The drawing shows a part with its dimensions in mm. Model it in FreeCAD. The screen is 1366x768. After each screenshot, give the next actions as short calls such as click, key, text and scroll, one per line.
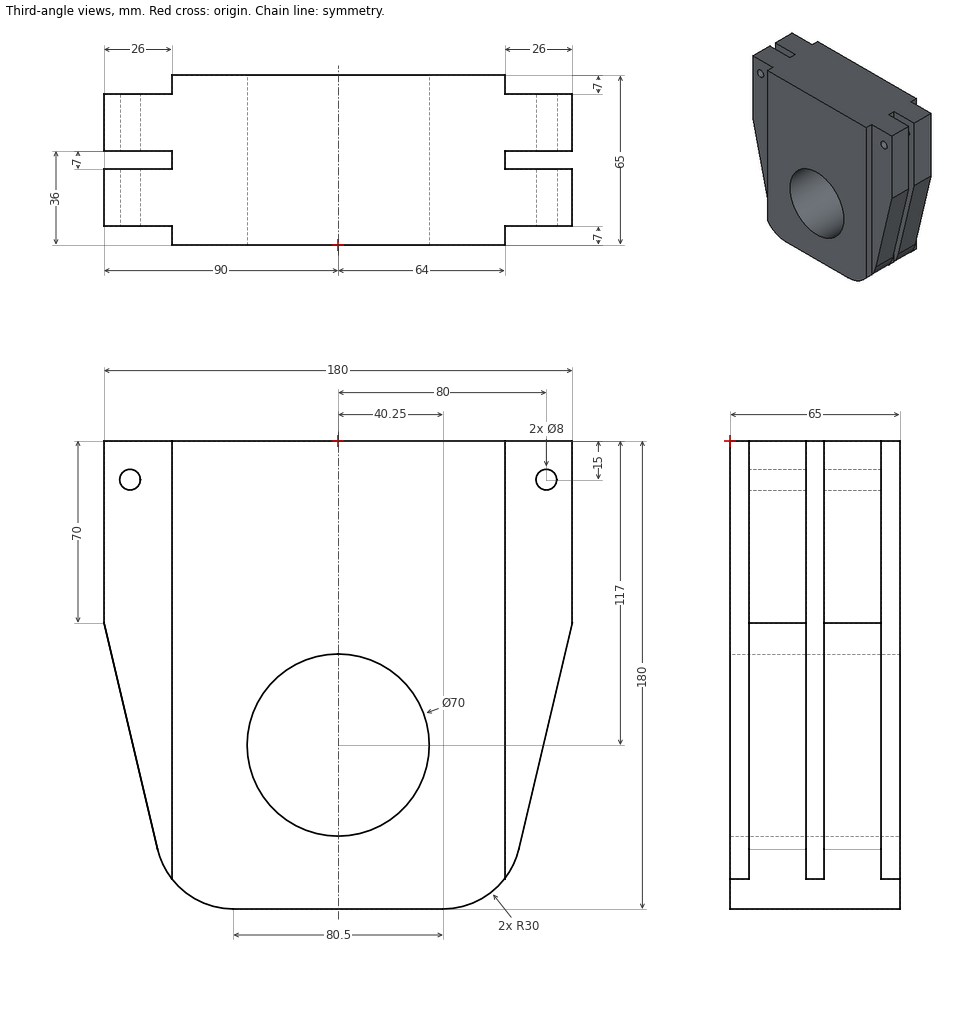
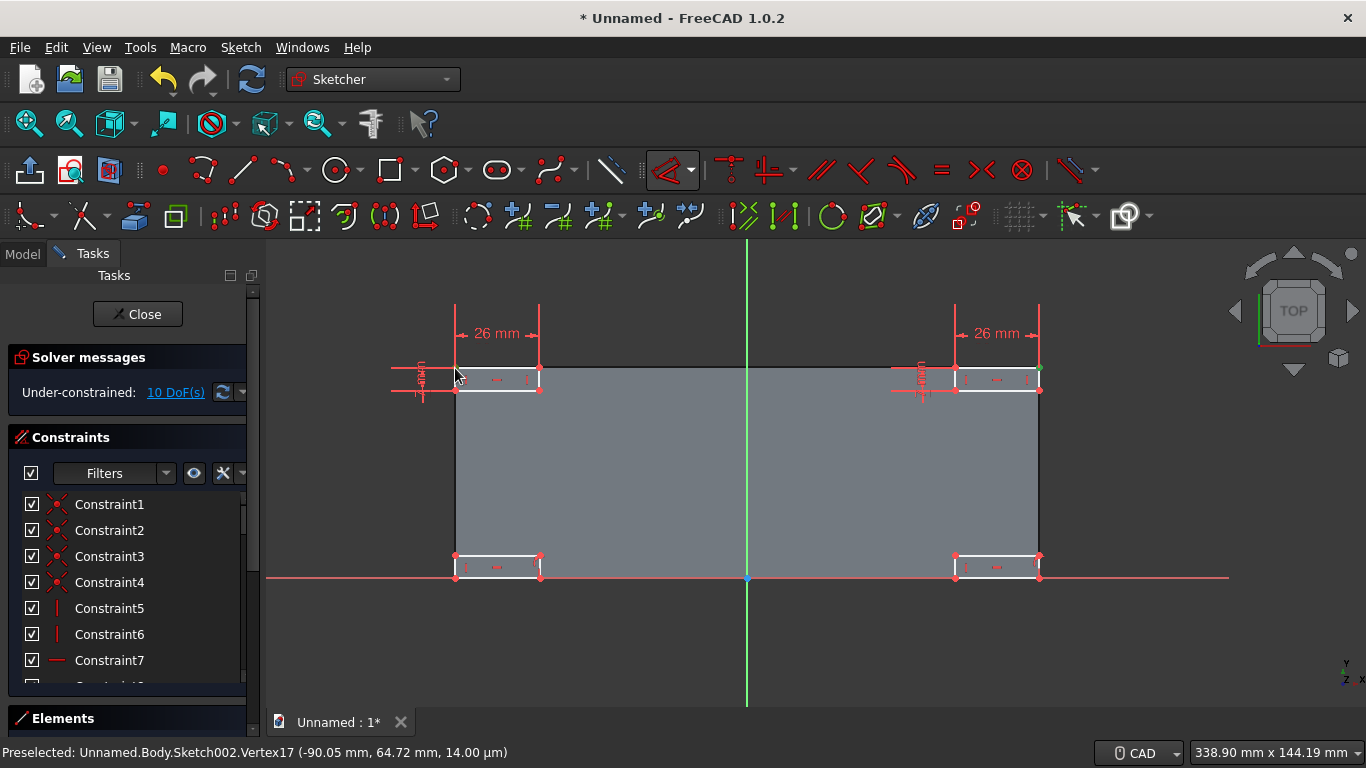
click(747, 650)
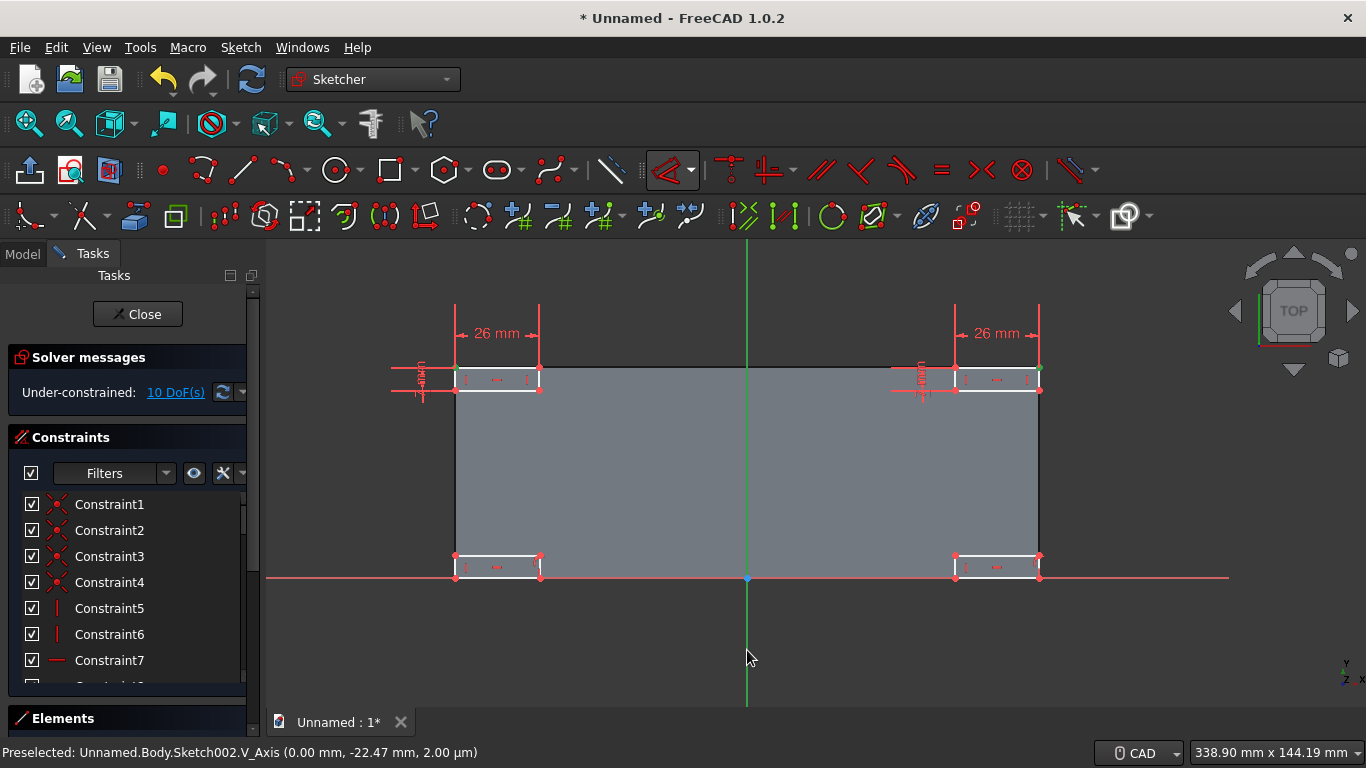
click(982, 170)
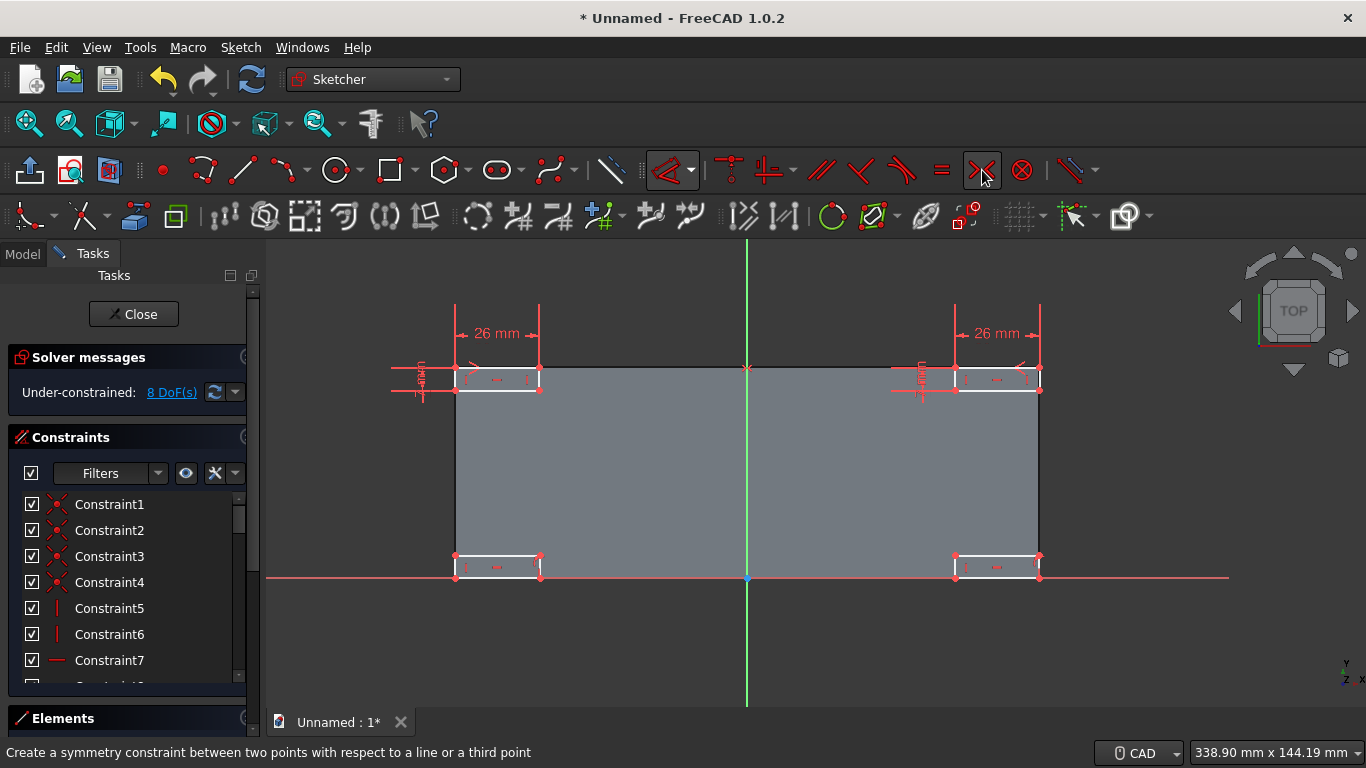
click(1039, 556)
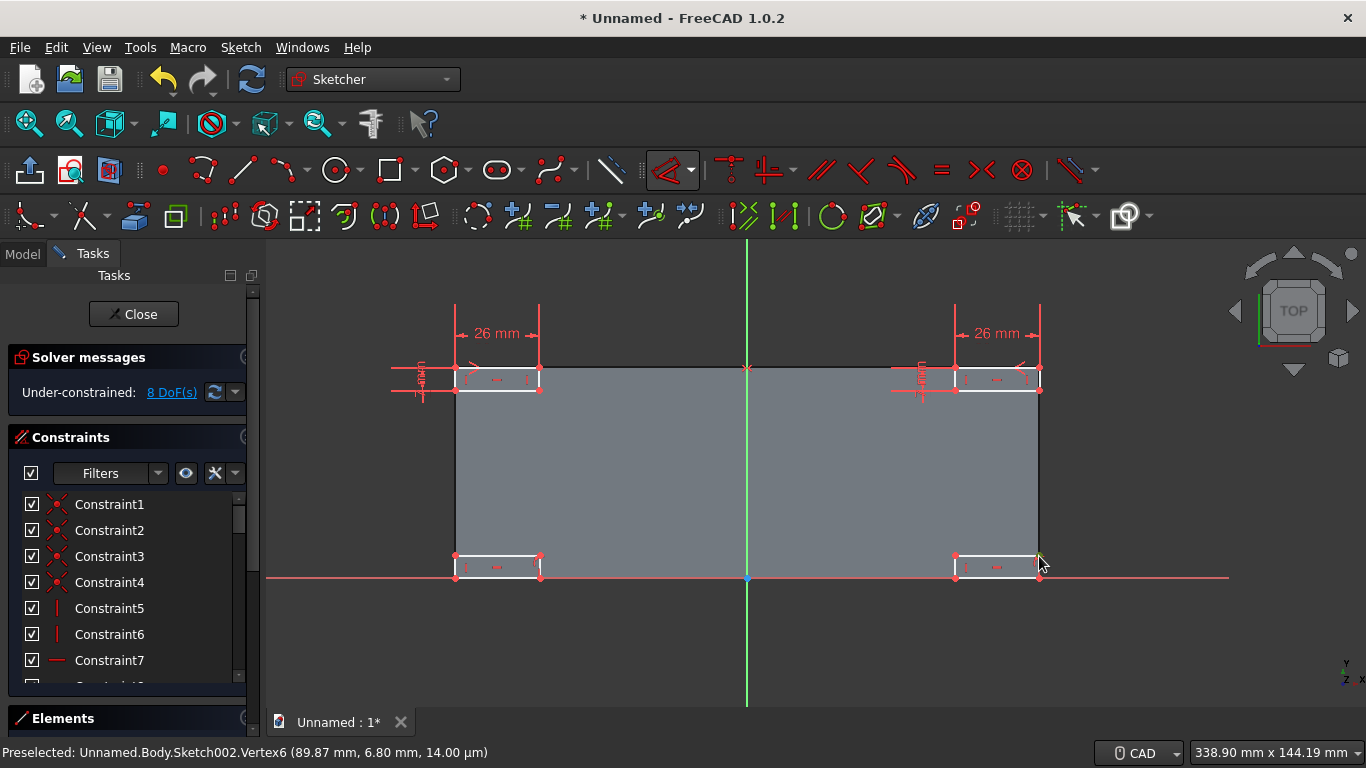
click(455, 556)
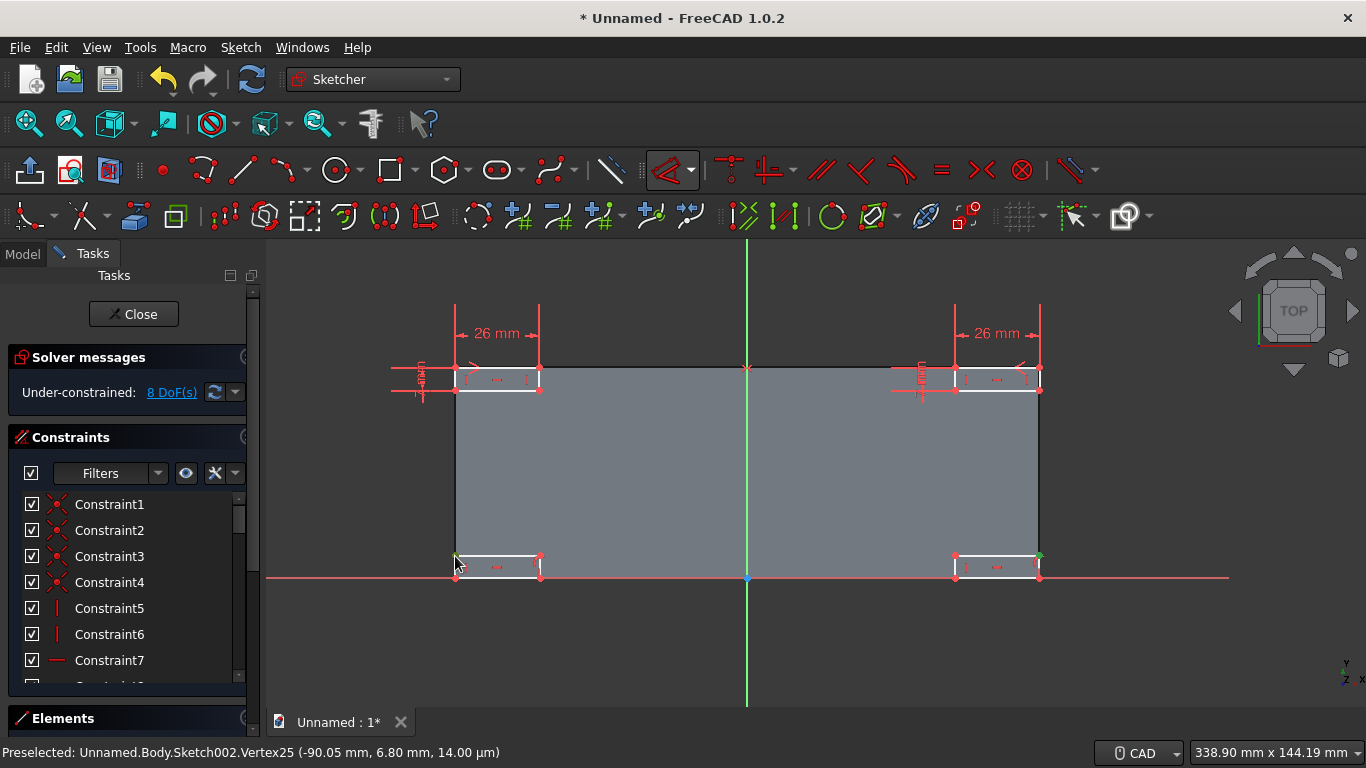
click(747, 650)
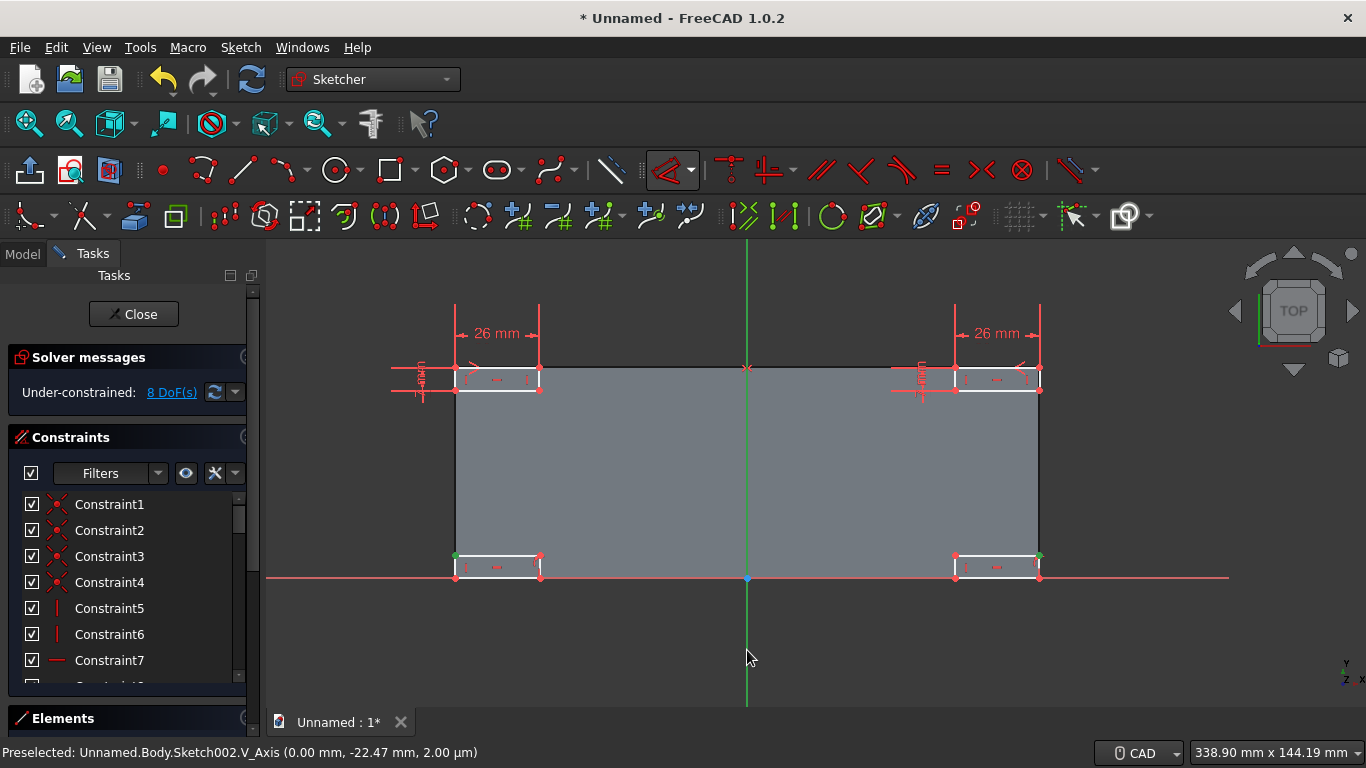
click(982, 170)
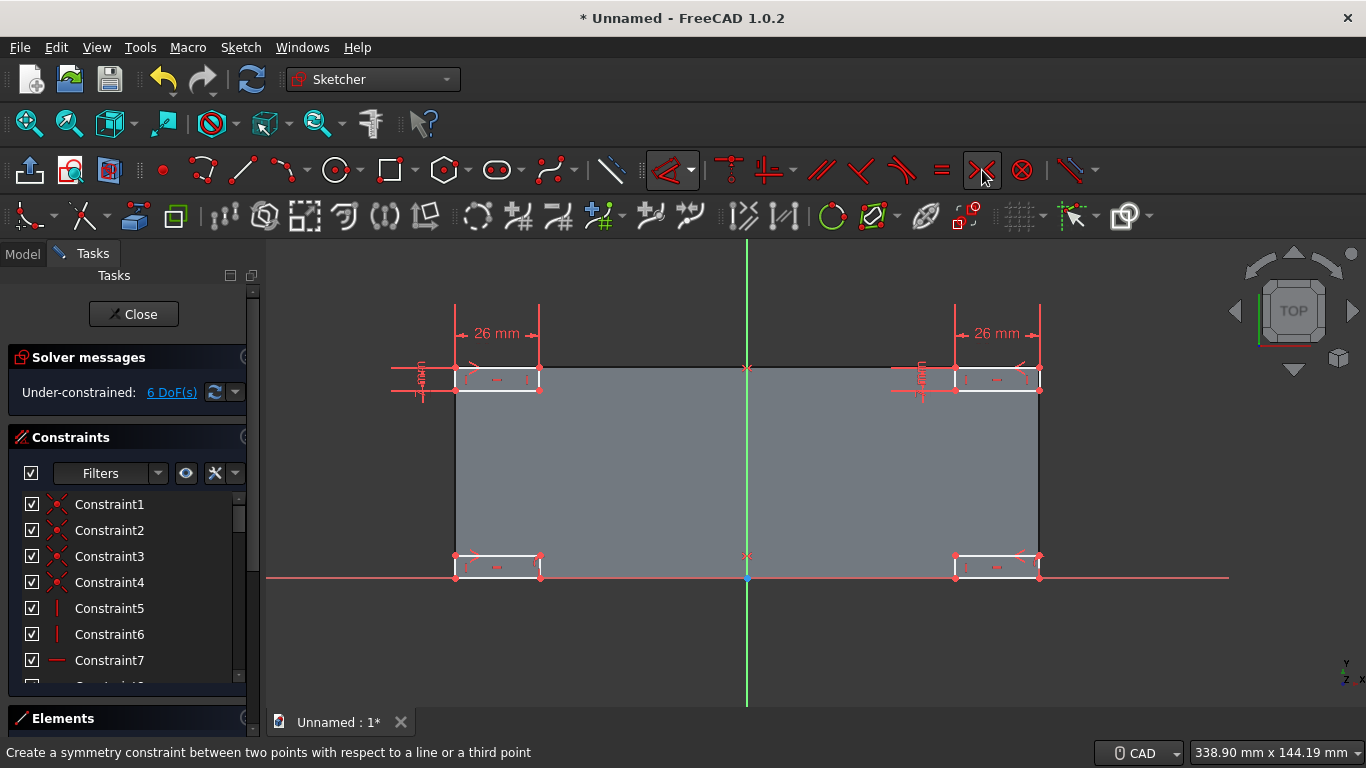
scroll(955, 567, up, 3)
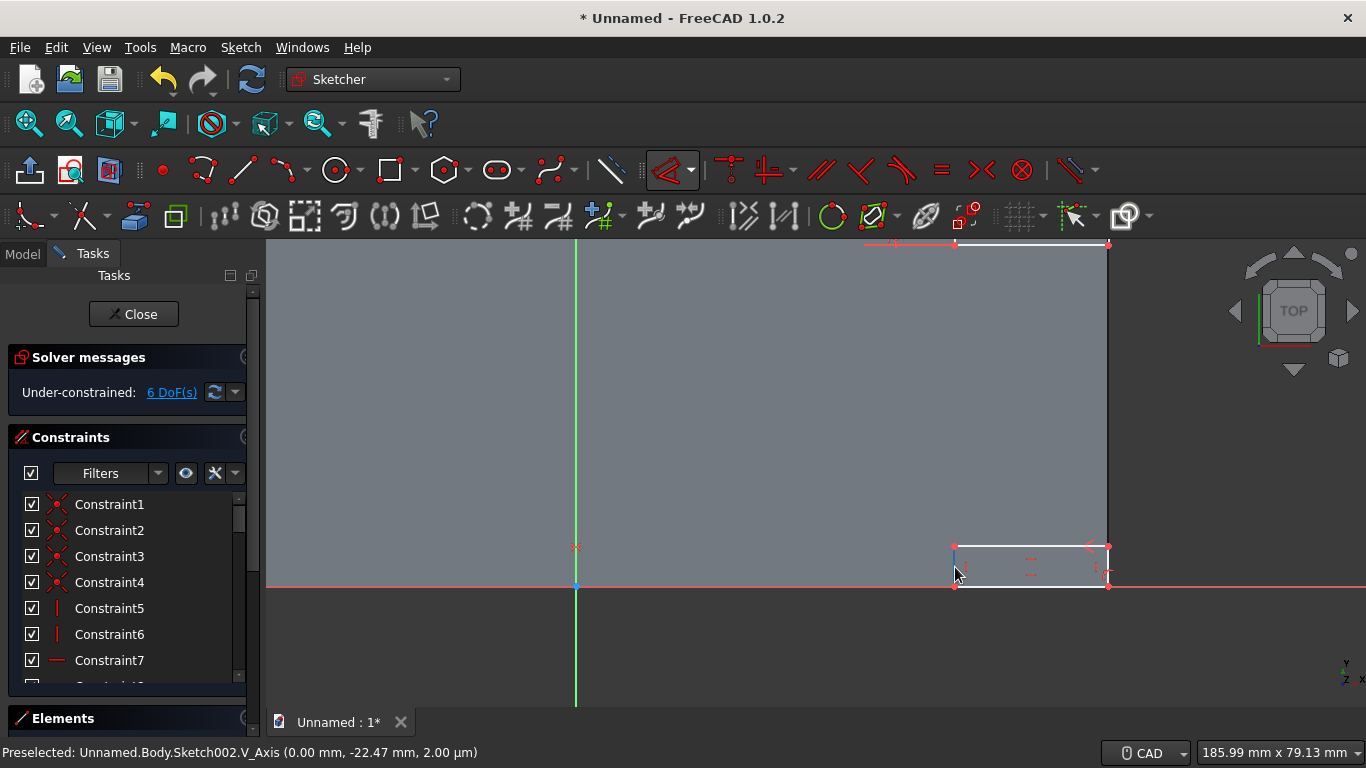
click(954, 566)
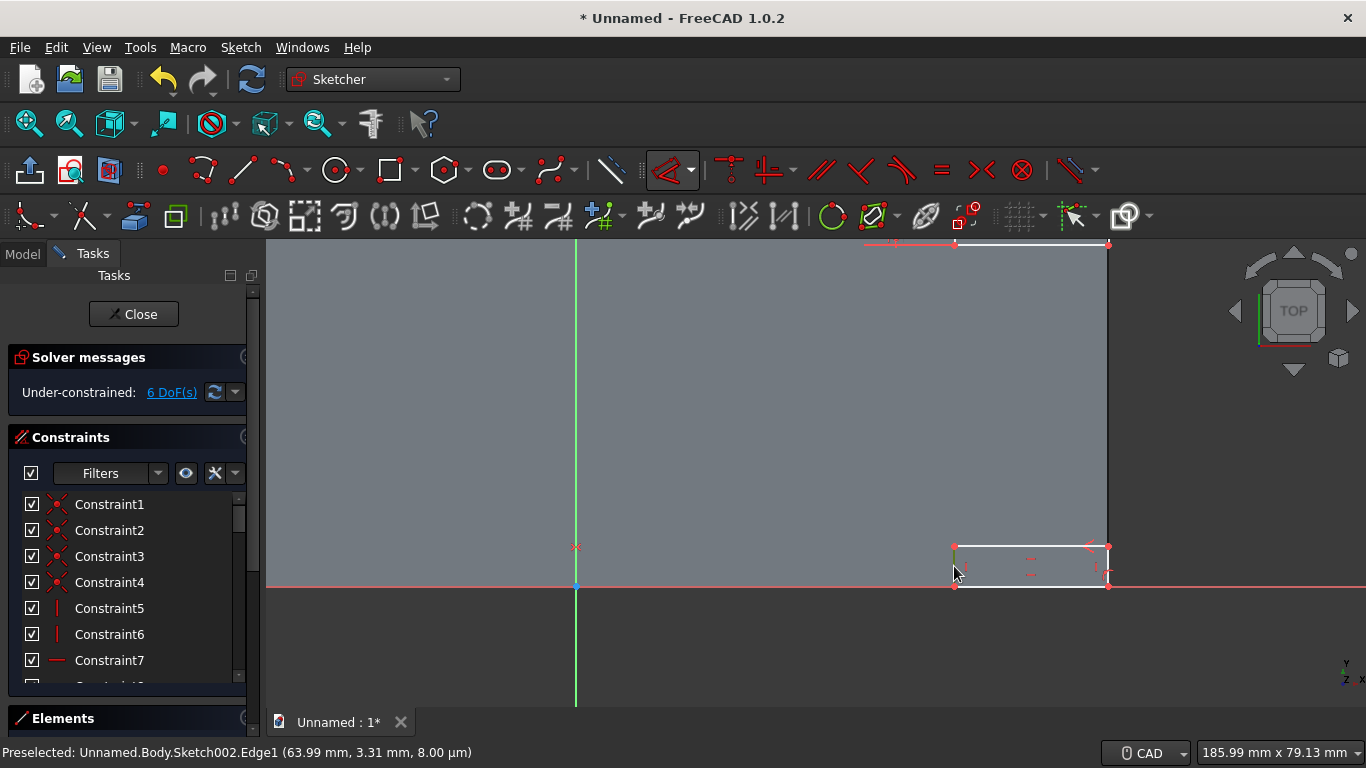
click(694, 170)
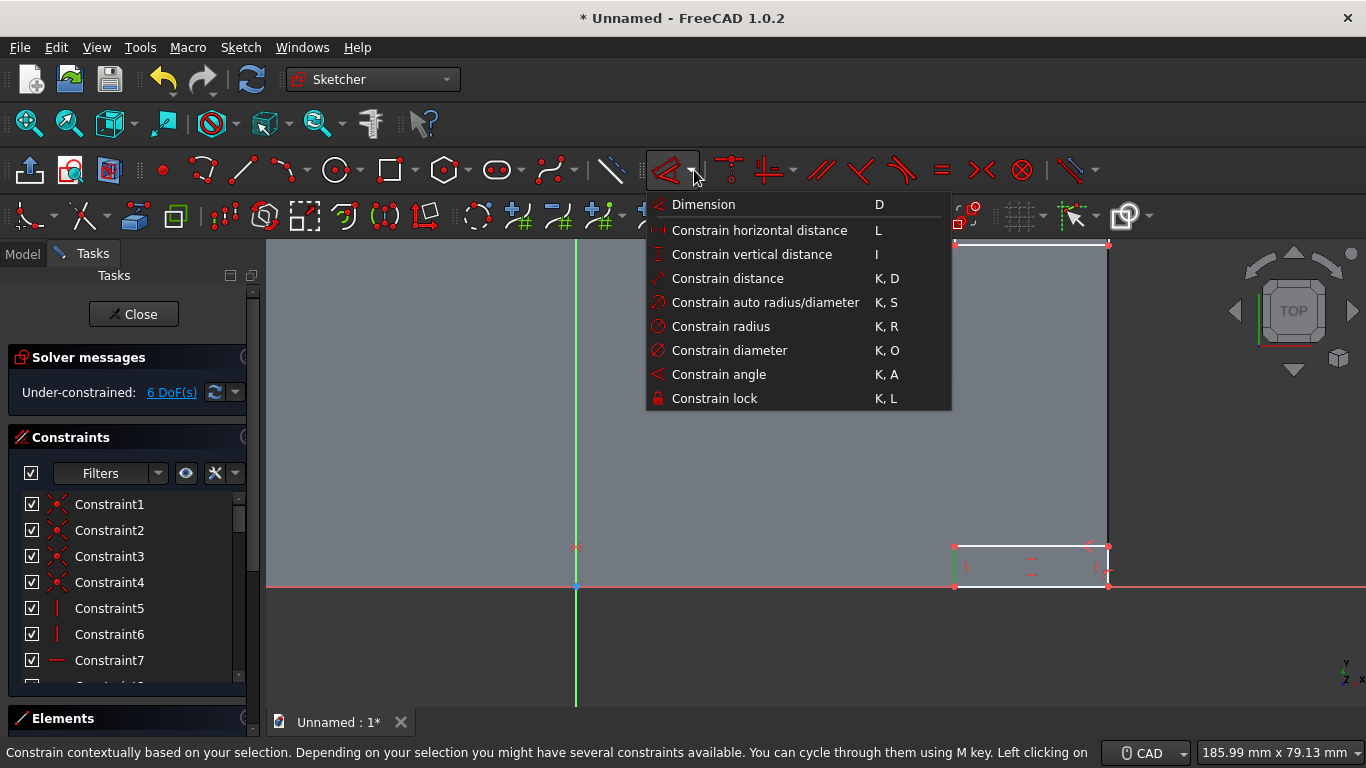
click(799, 254)